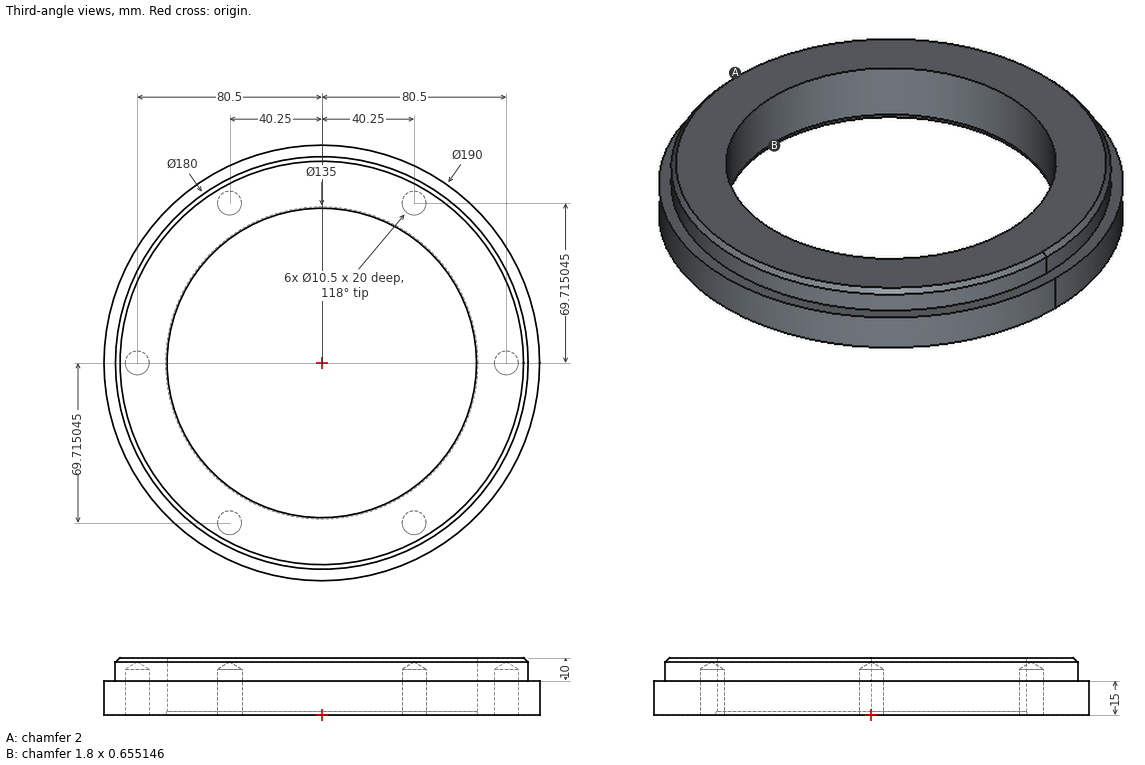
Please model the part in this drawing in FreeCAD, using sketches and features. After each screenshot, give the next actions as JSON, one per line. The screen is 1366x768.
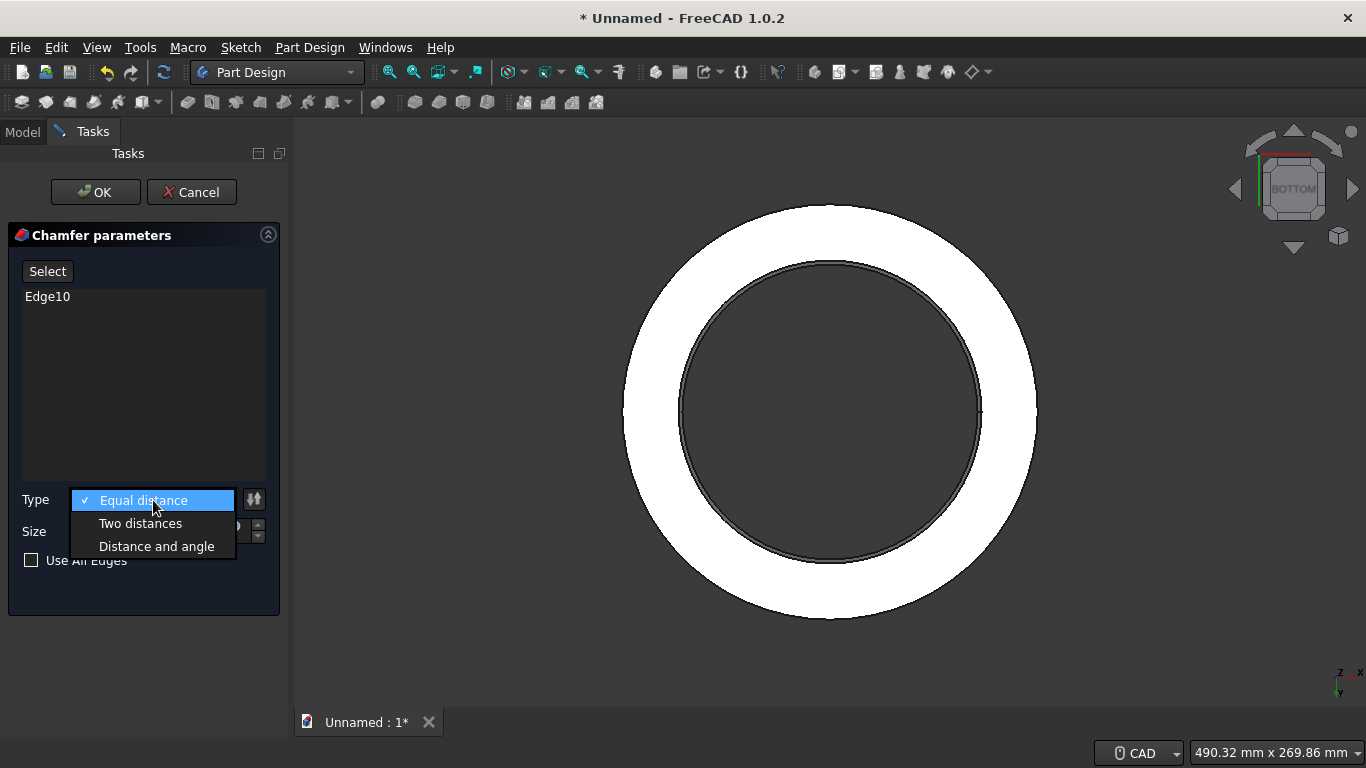
{"action": "left_click", "coordinate": [152, 524]}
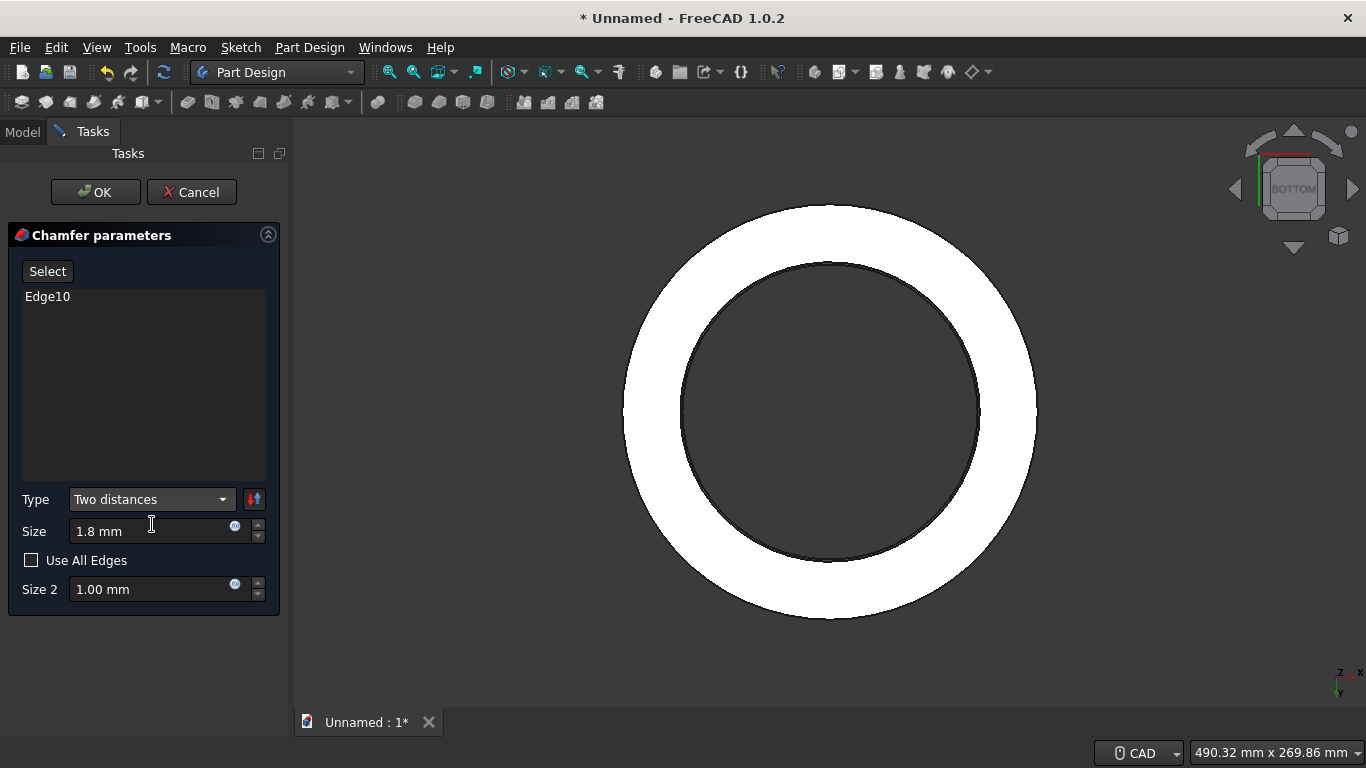
{"action": "triple_click", "coordinate": [160, 589]}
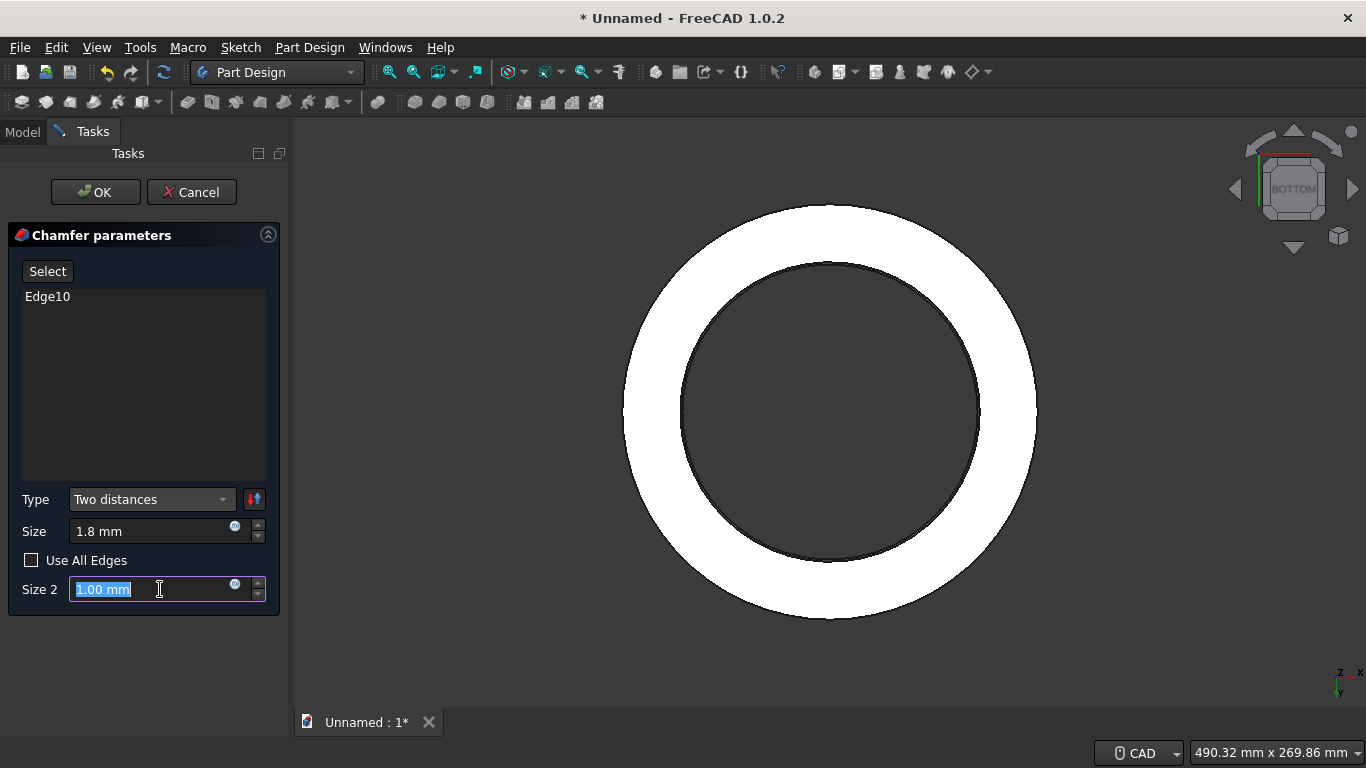
{"action": "type", "text": "0.655146"}
{"action": "key", "text": "Tab"}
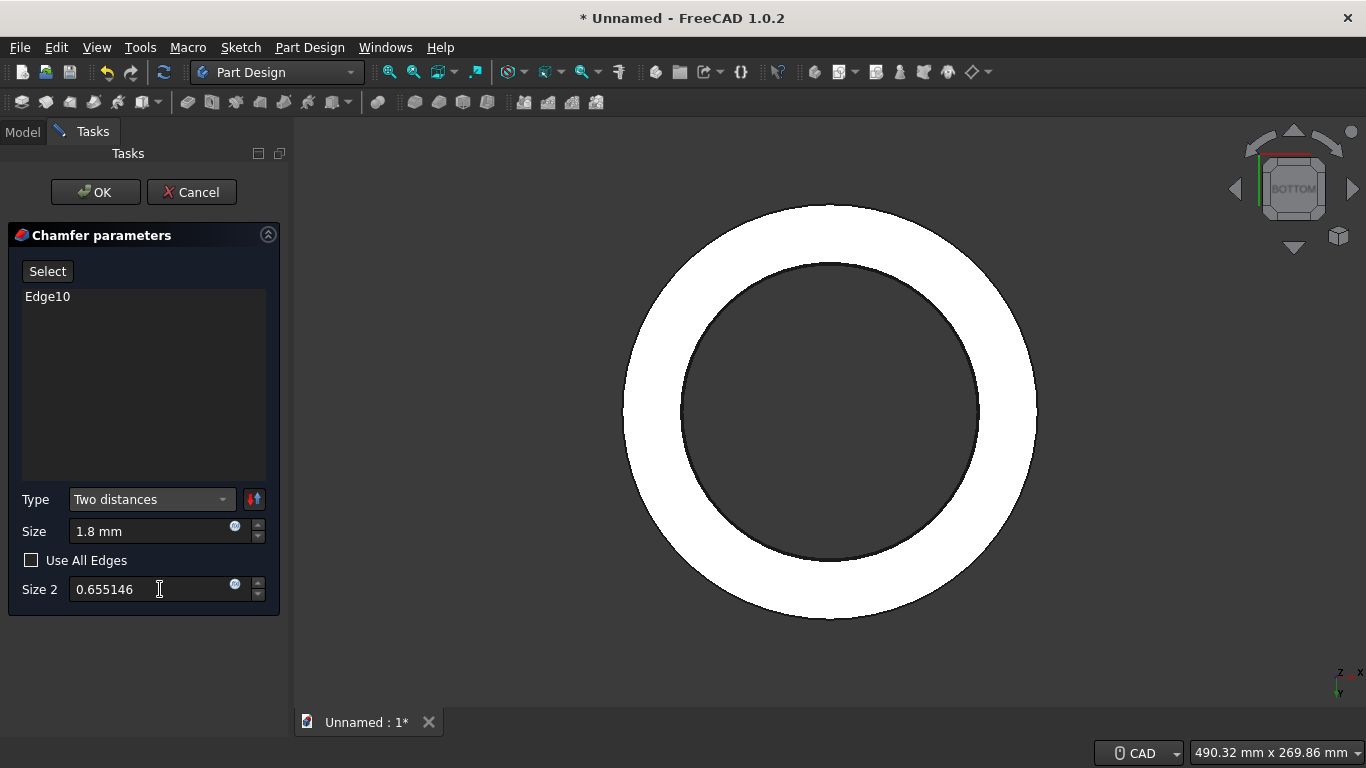
{"action": "left_click", "coordinate": [96, 192]}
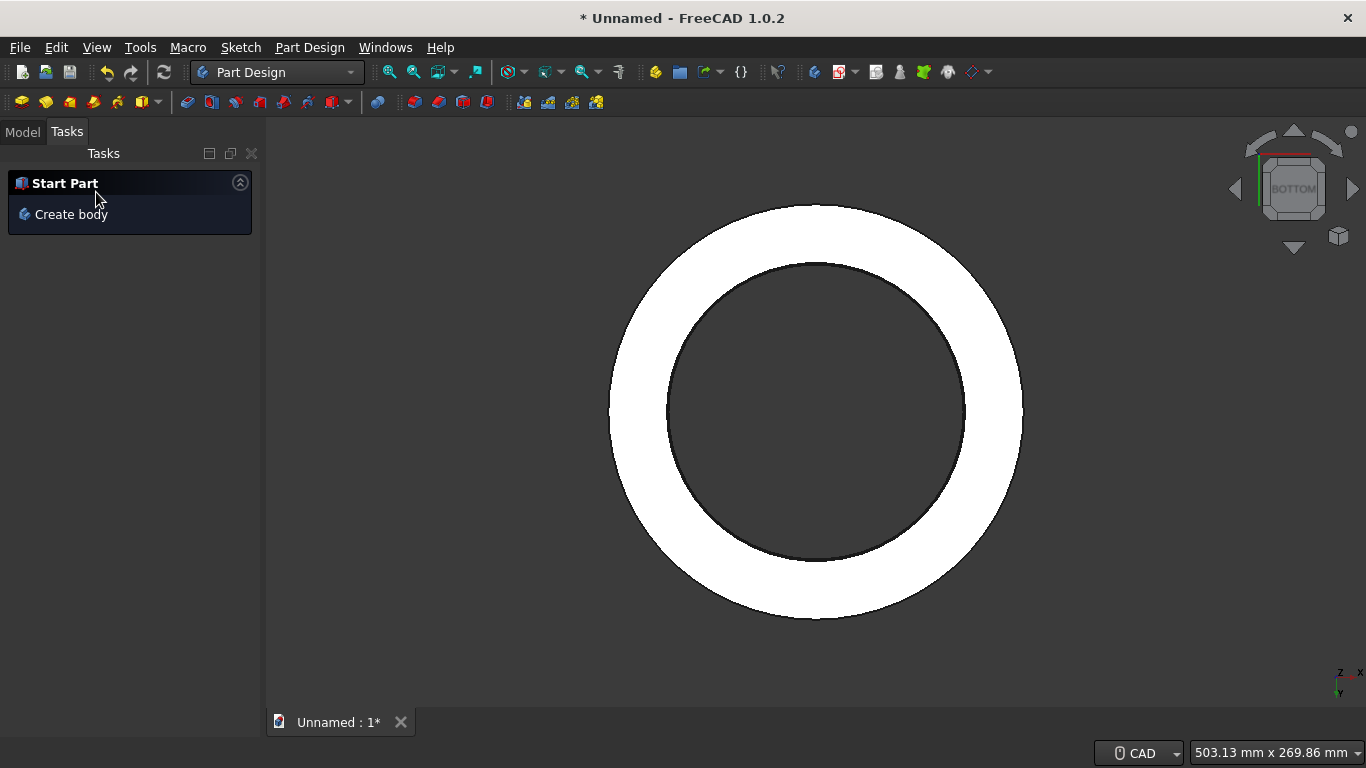
{"action": "left_click", "coordinate": [816, 233]}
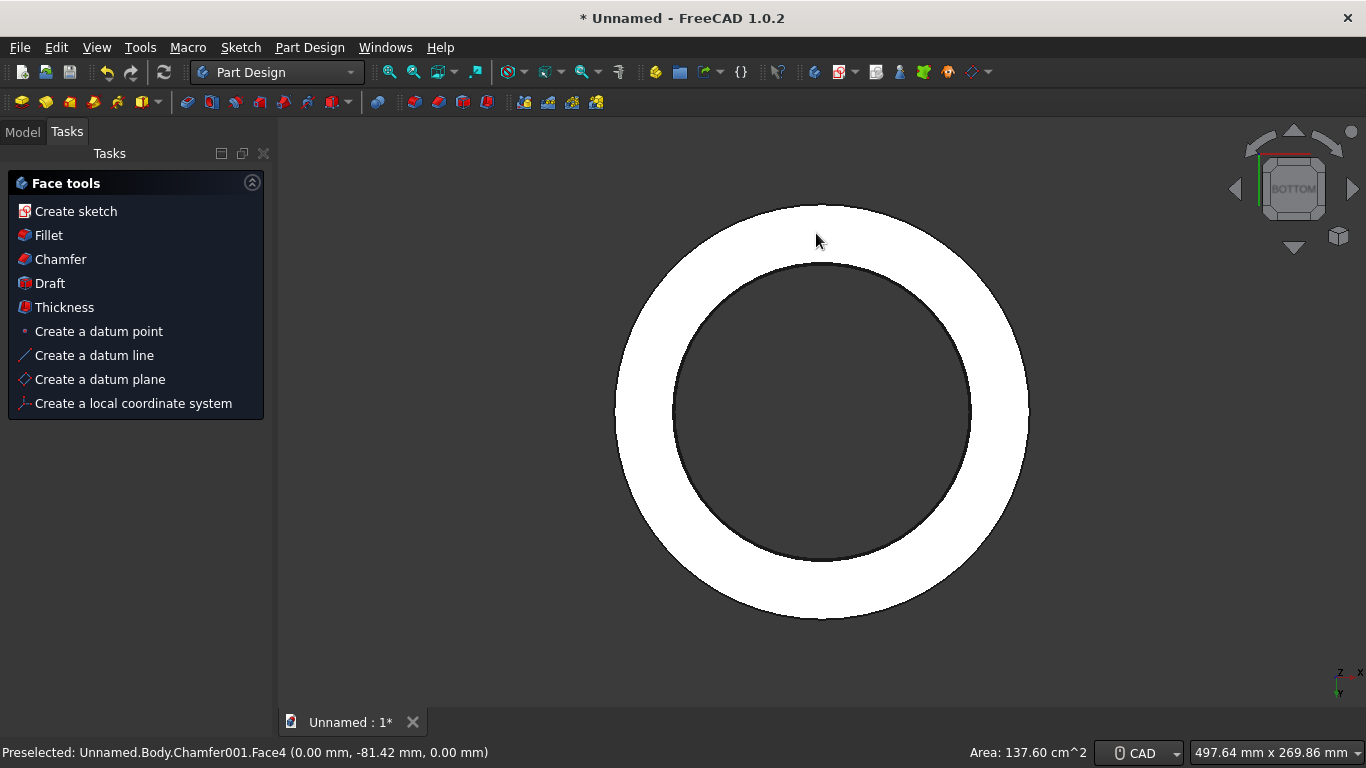
{"action": "left_click", "coordinate": [840, 72]}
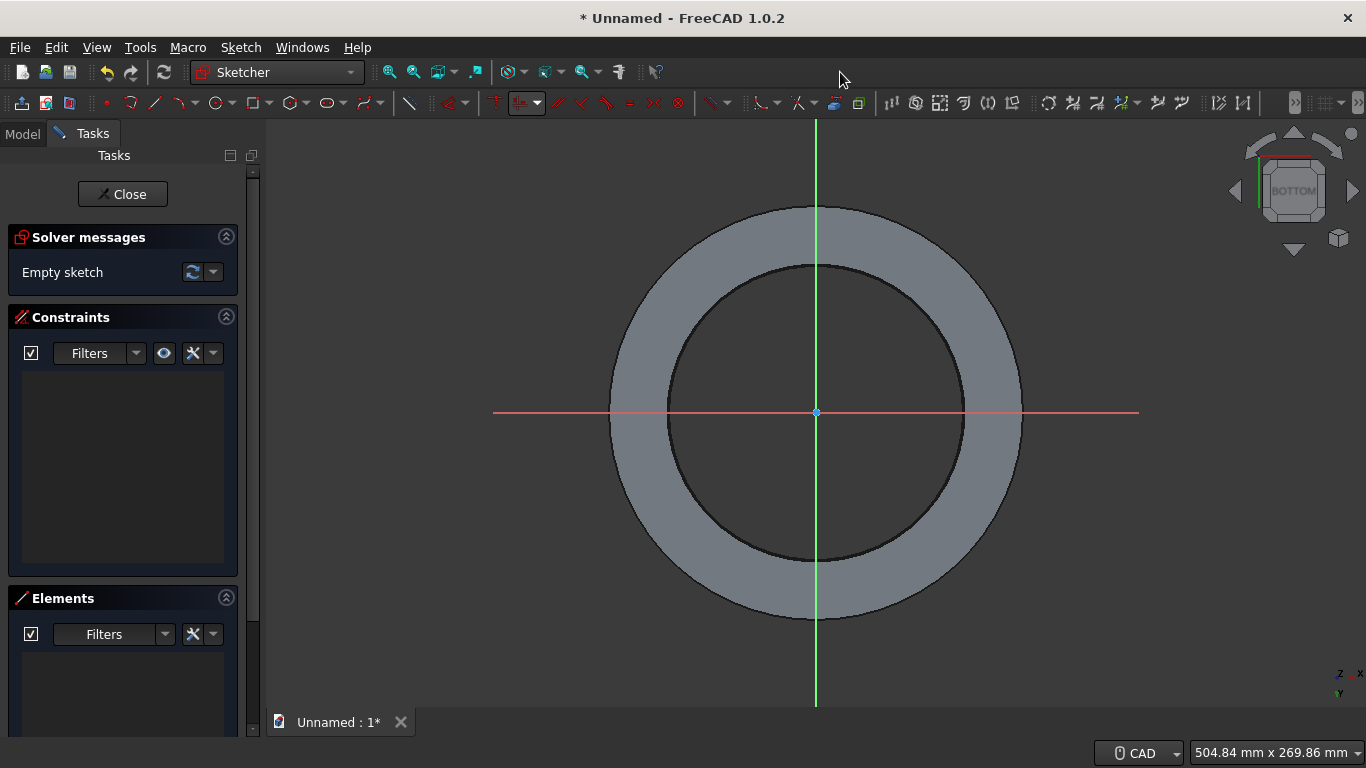
{"action": "left_click", "coordinate": [216, 104]}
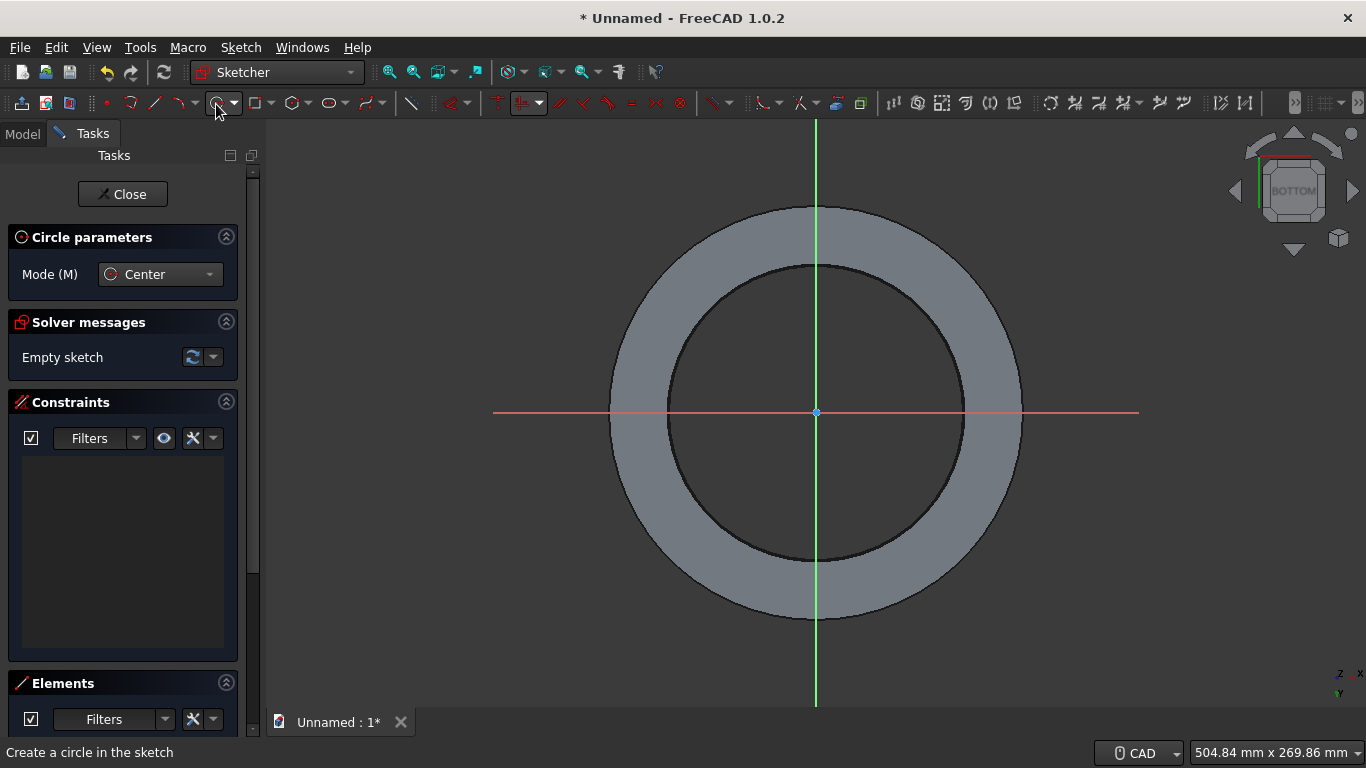
{"action": "scroll", "coordinate": [904, 565], "scroll_direction": "up", "scroll_amount": 4}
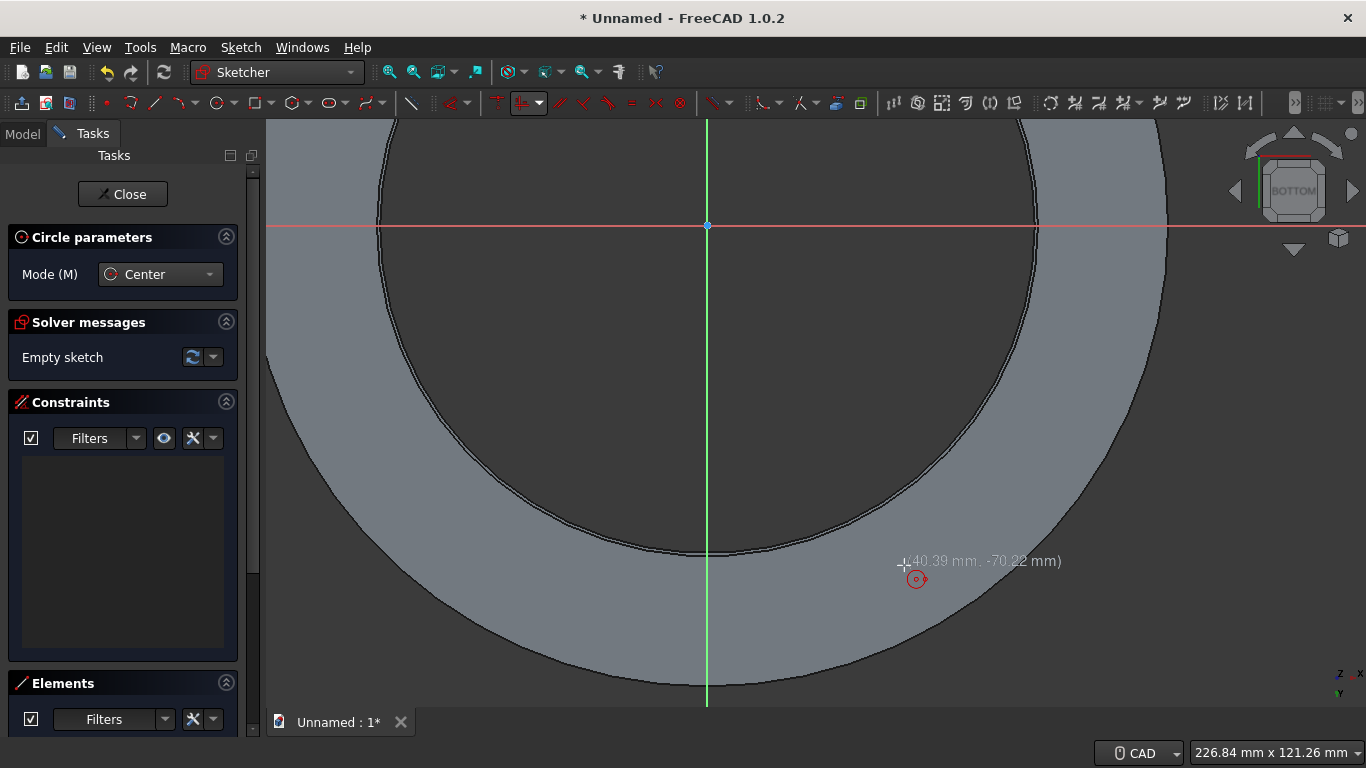
{"action": "left_click", "coordinate": [903, 564]}
{"action": "left_click", "coordinate": [921, 546]}